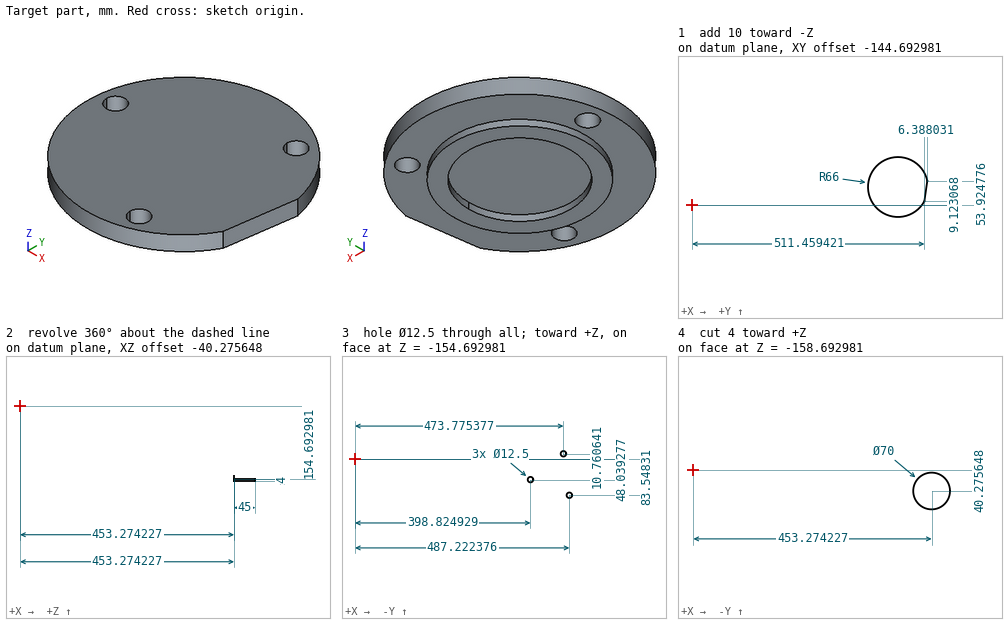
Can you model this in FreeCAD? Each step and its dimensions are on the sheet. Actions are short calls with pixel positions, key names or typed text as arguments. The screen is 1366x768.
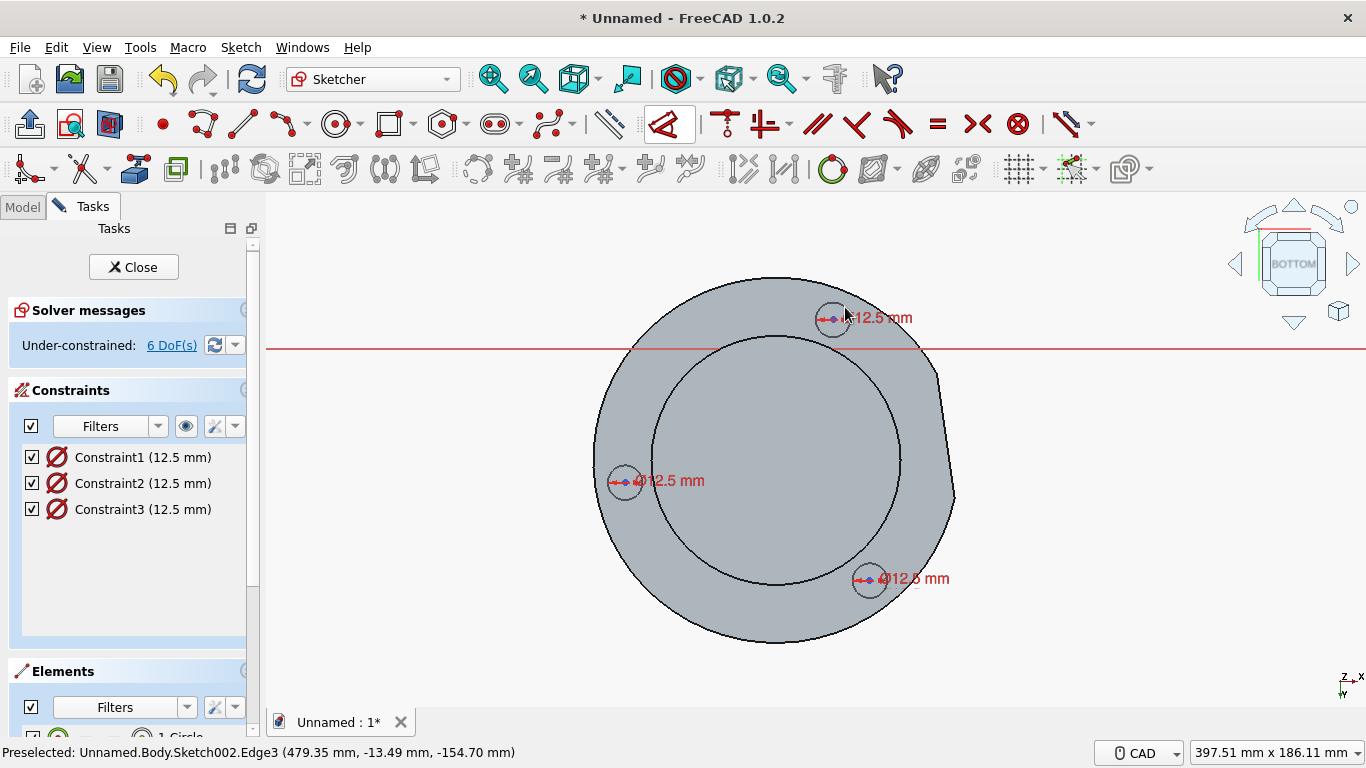
click(870, 581)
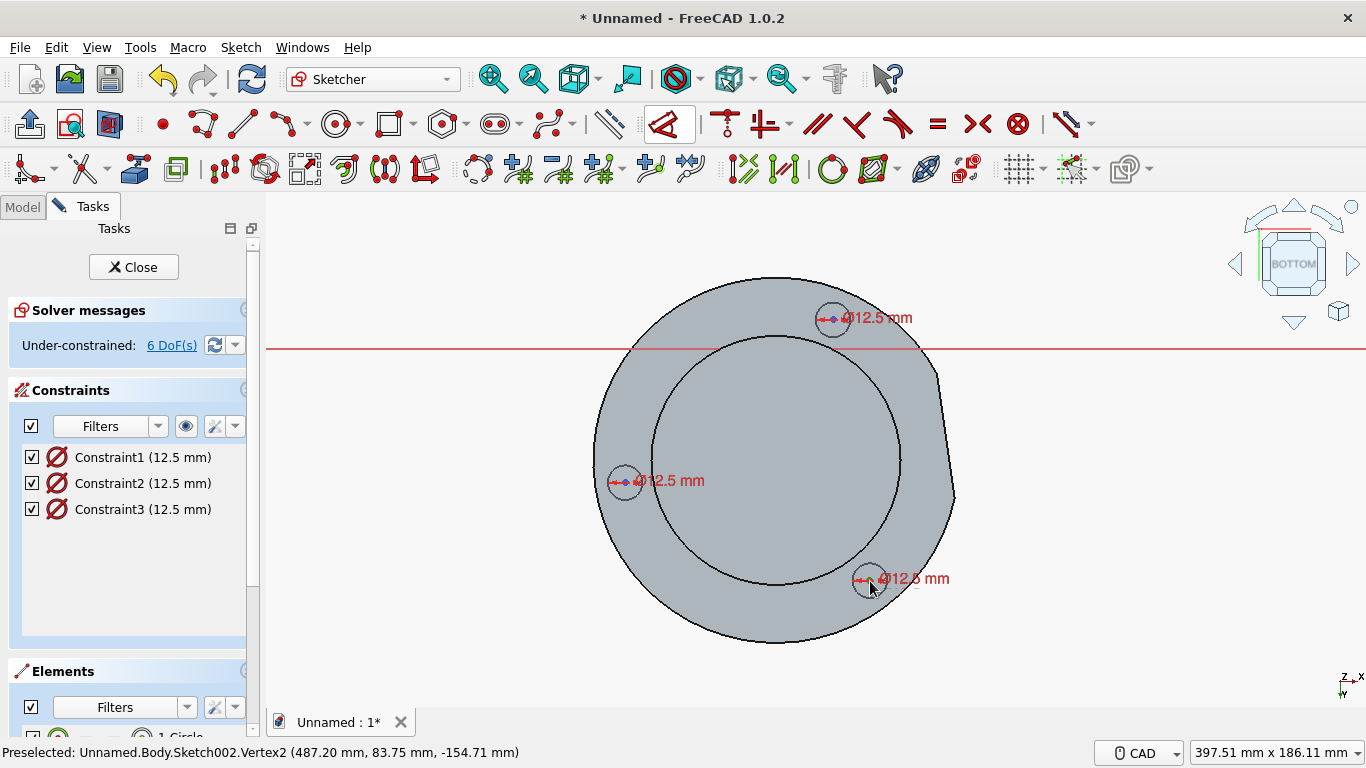
key(i)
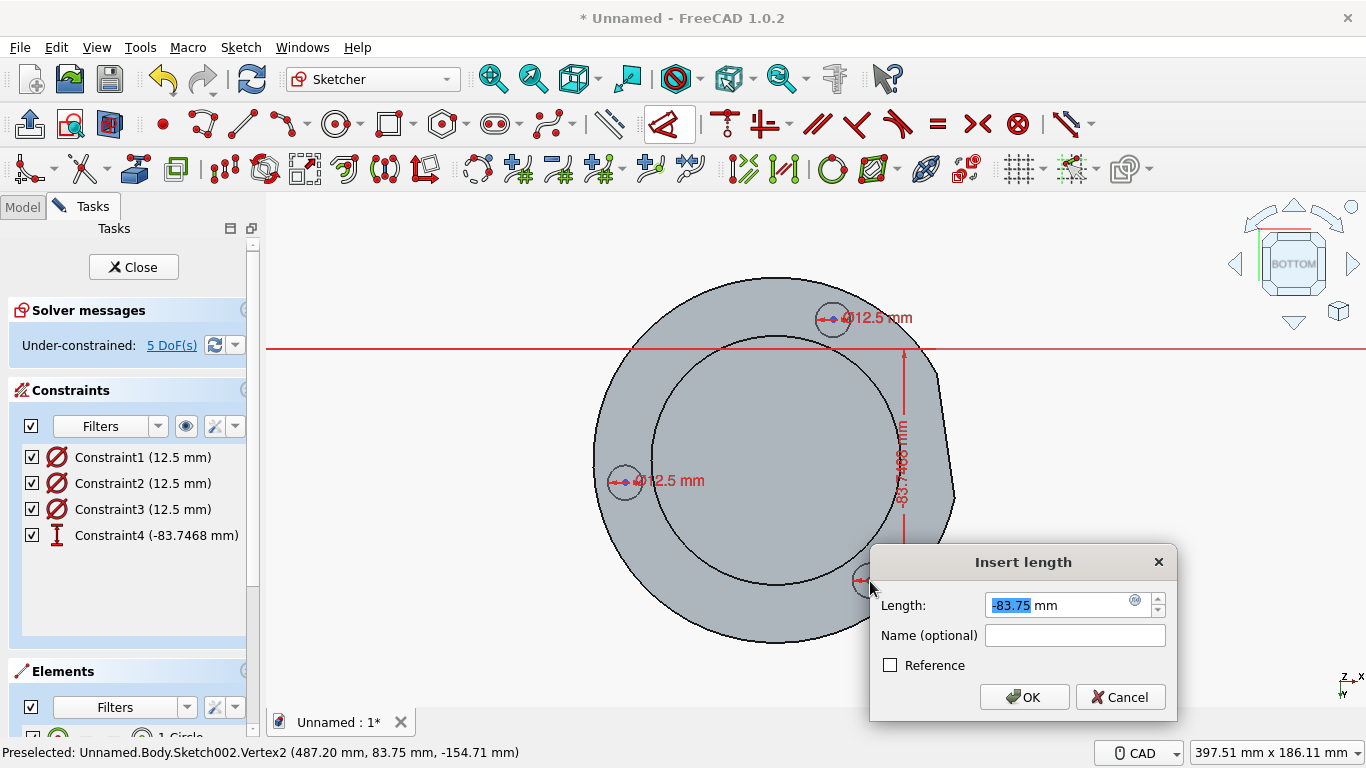
text(-83.54831)
key(Return)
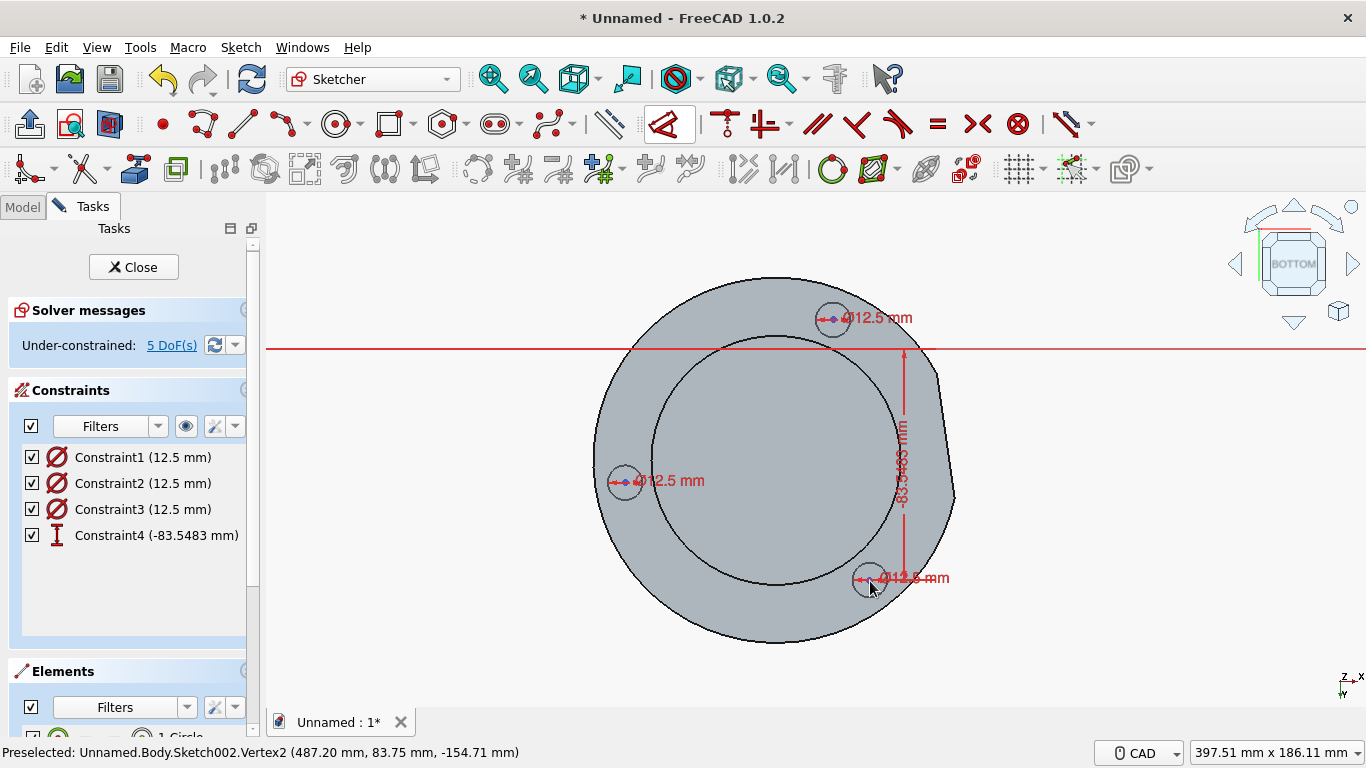
click(625, 483)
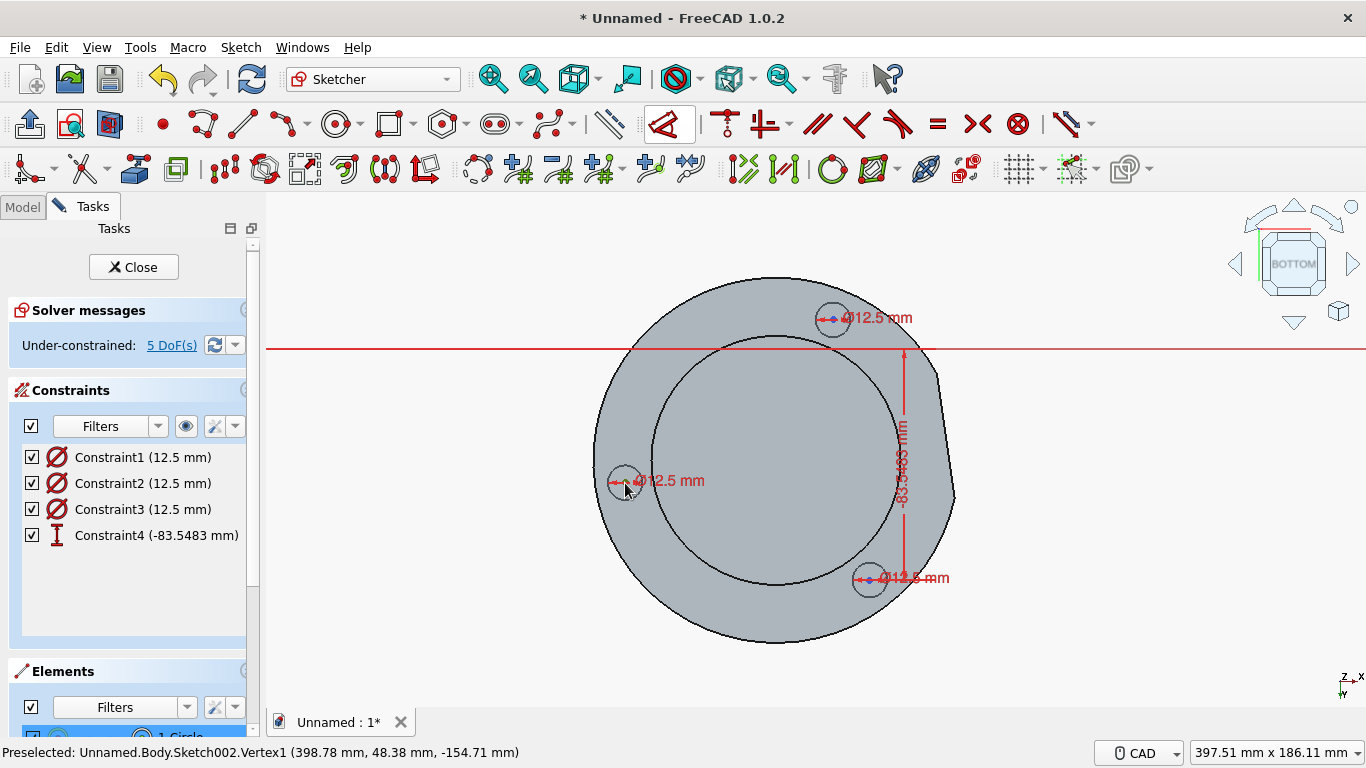
click(690, 124)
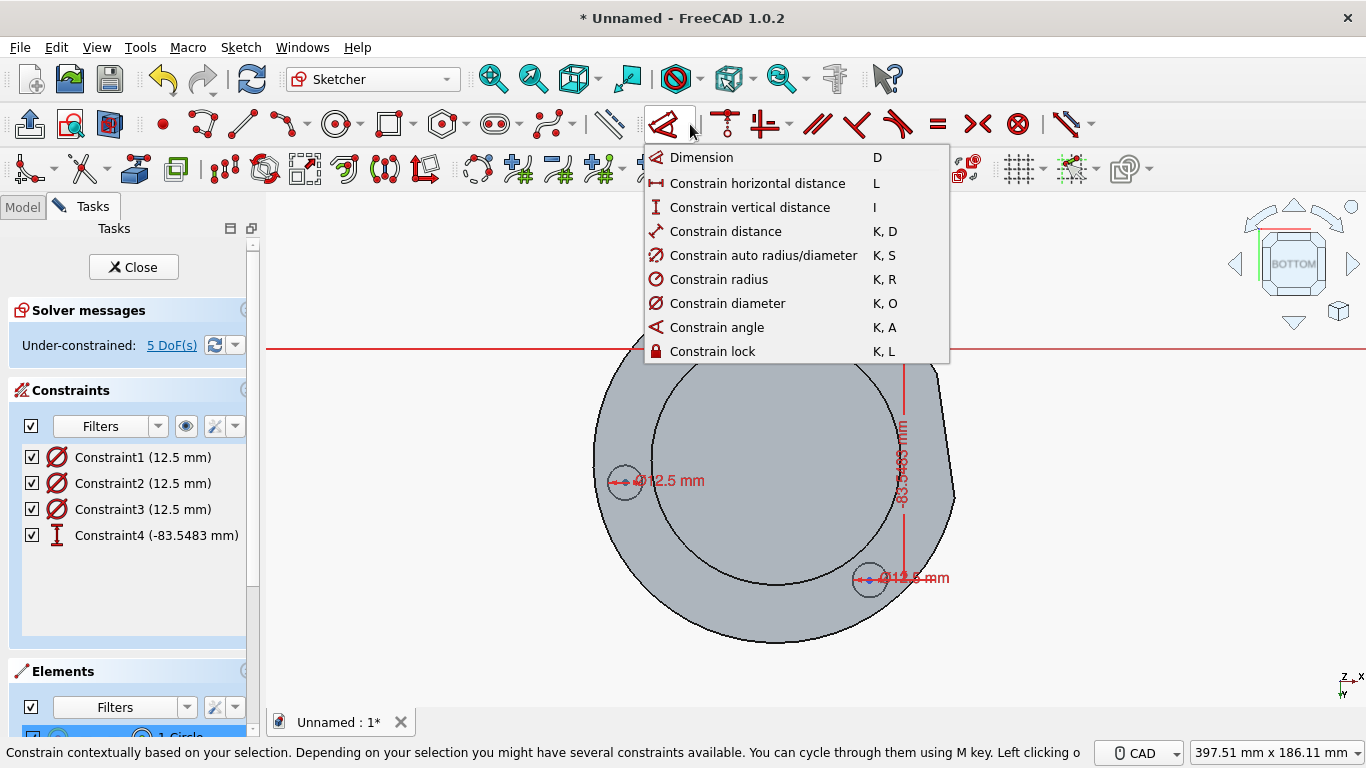
click(797, 207)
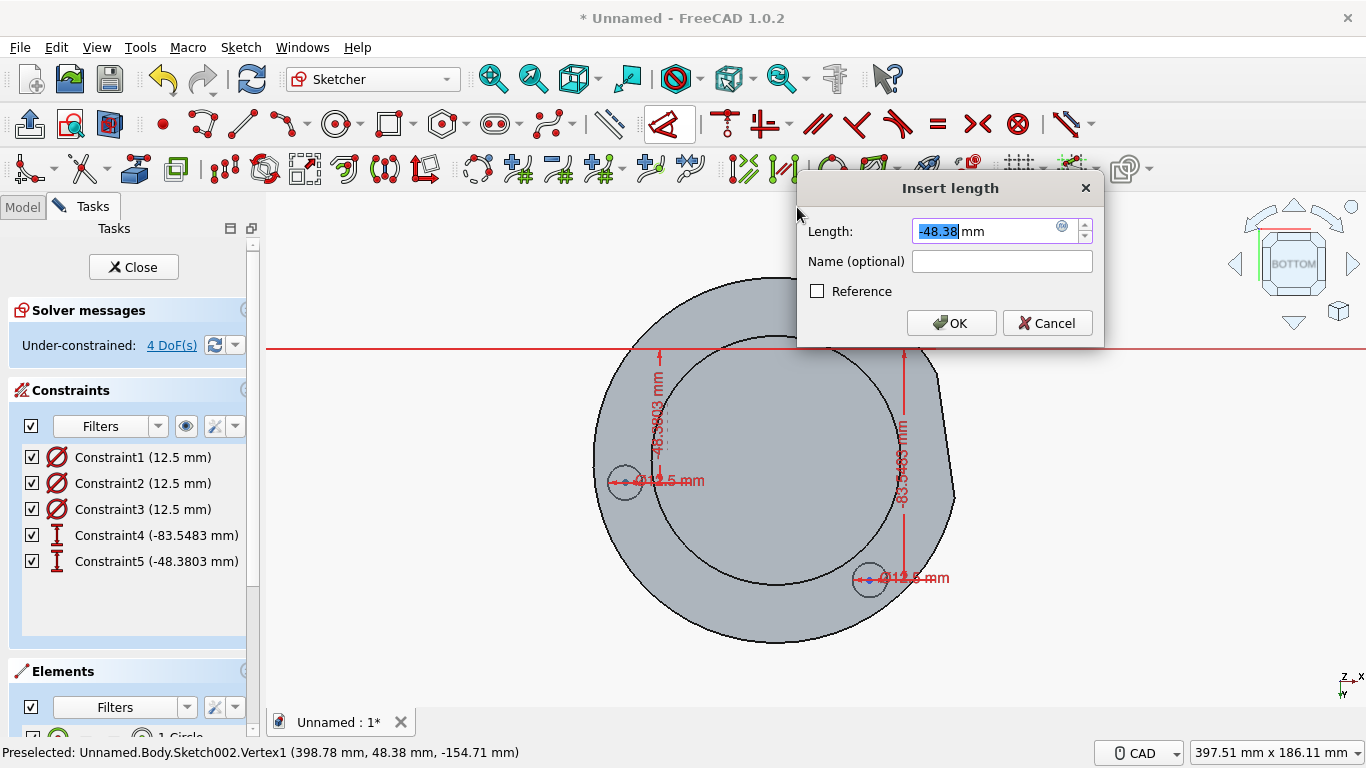
text(-48.039277)
key(Return)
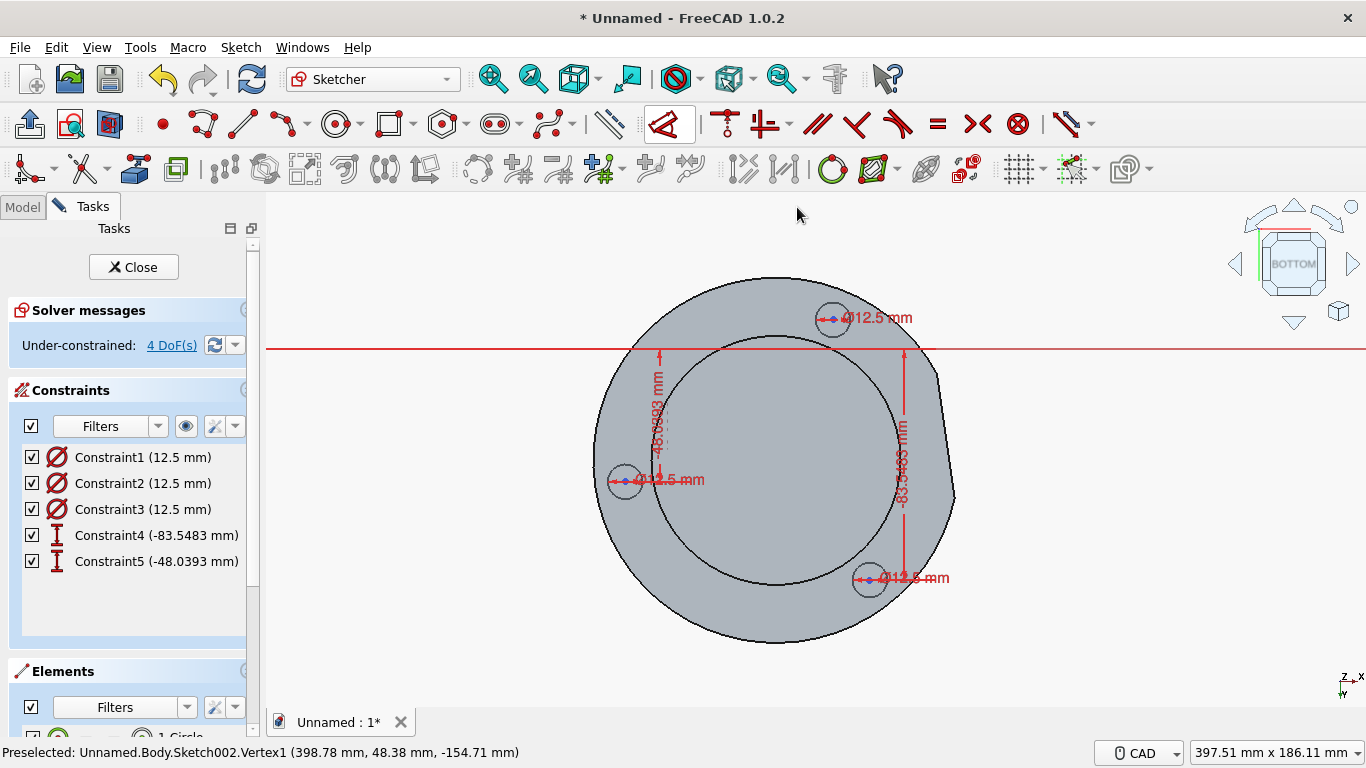
scroll(833, 320, up, 2)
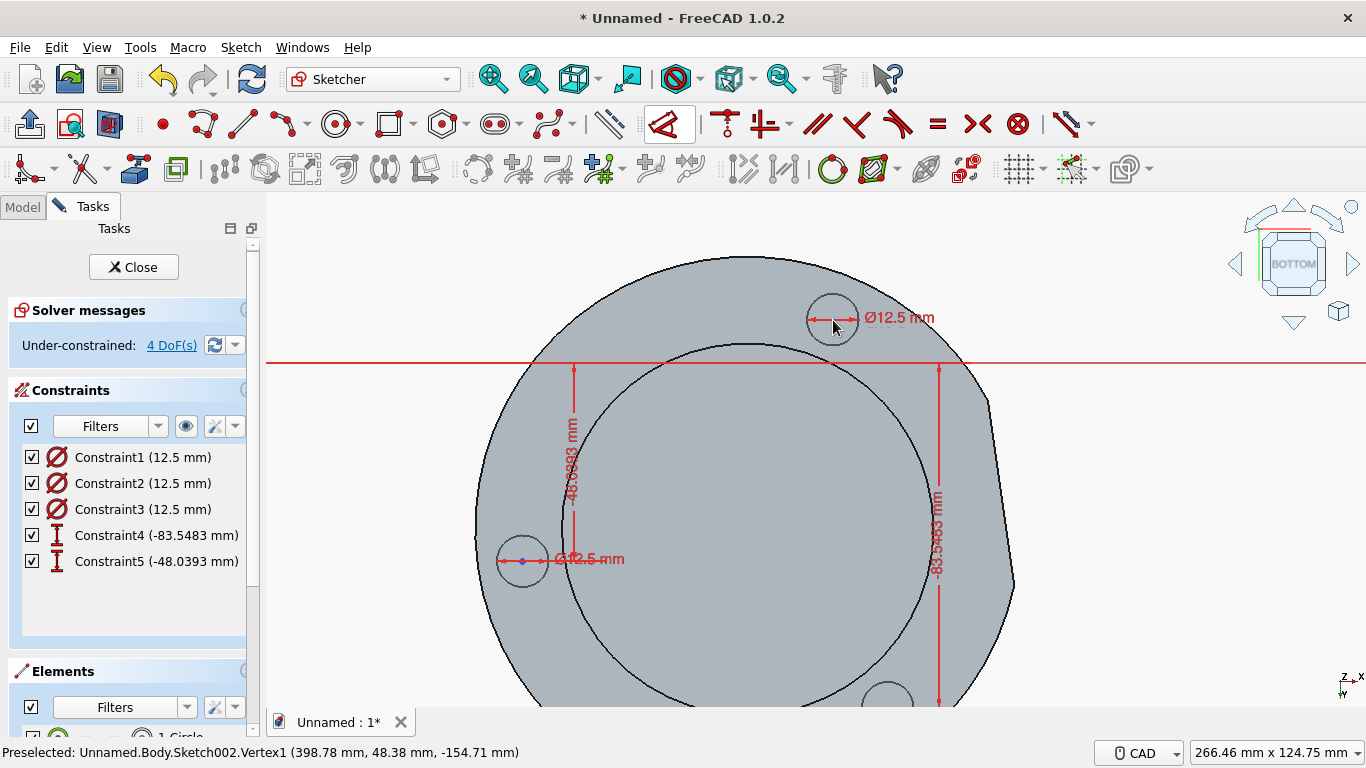
click(833, 320)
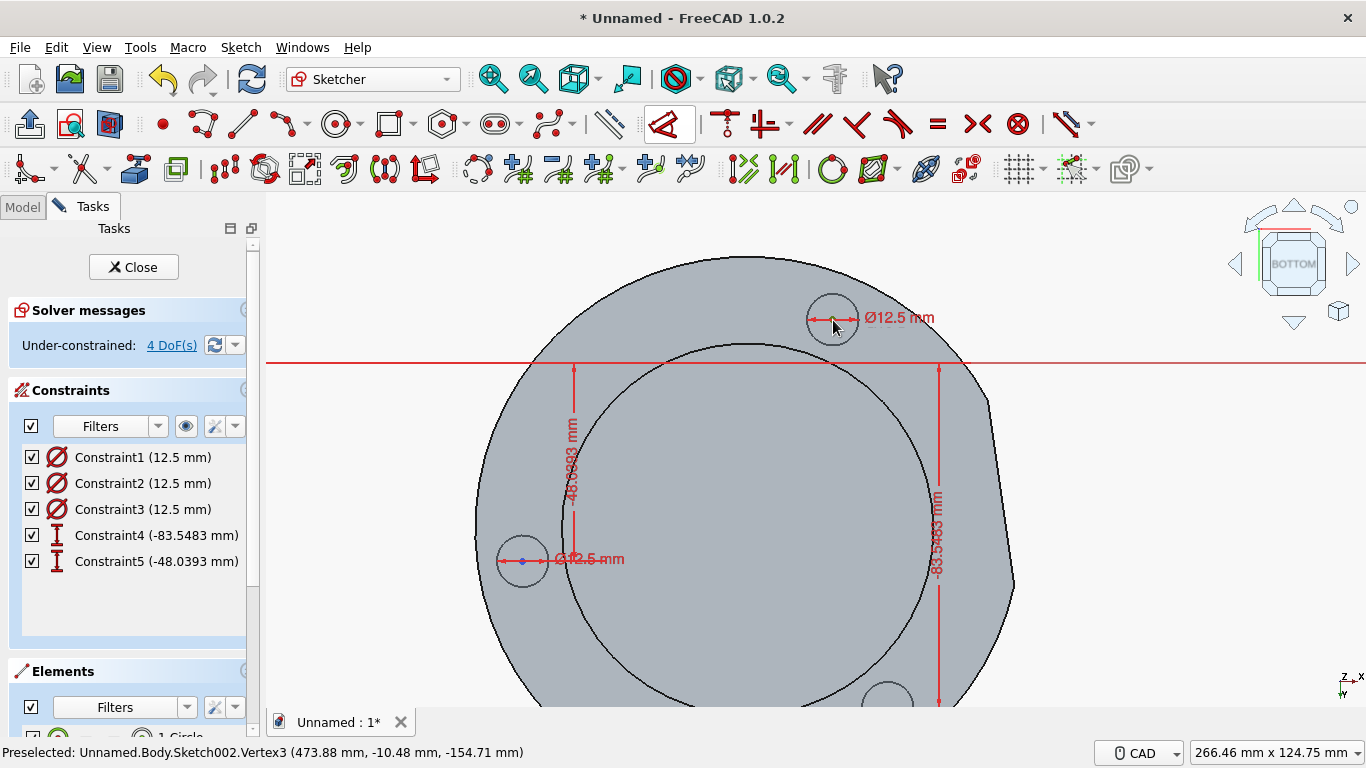
key(i)